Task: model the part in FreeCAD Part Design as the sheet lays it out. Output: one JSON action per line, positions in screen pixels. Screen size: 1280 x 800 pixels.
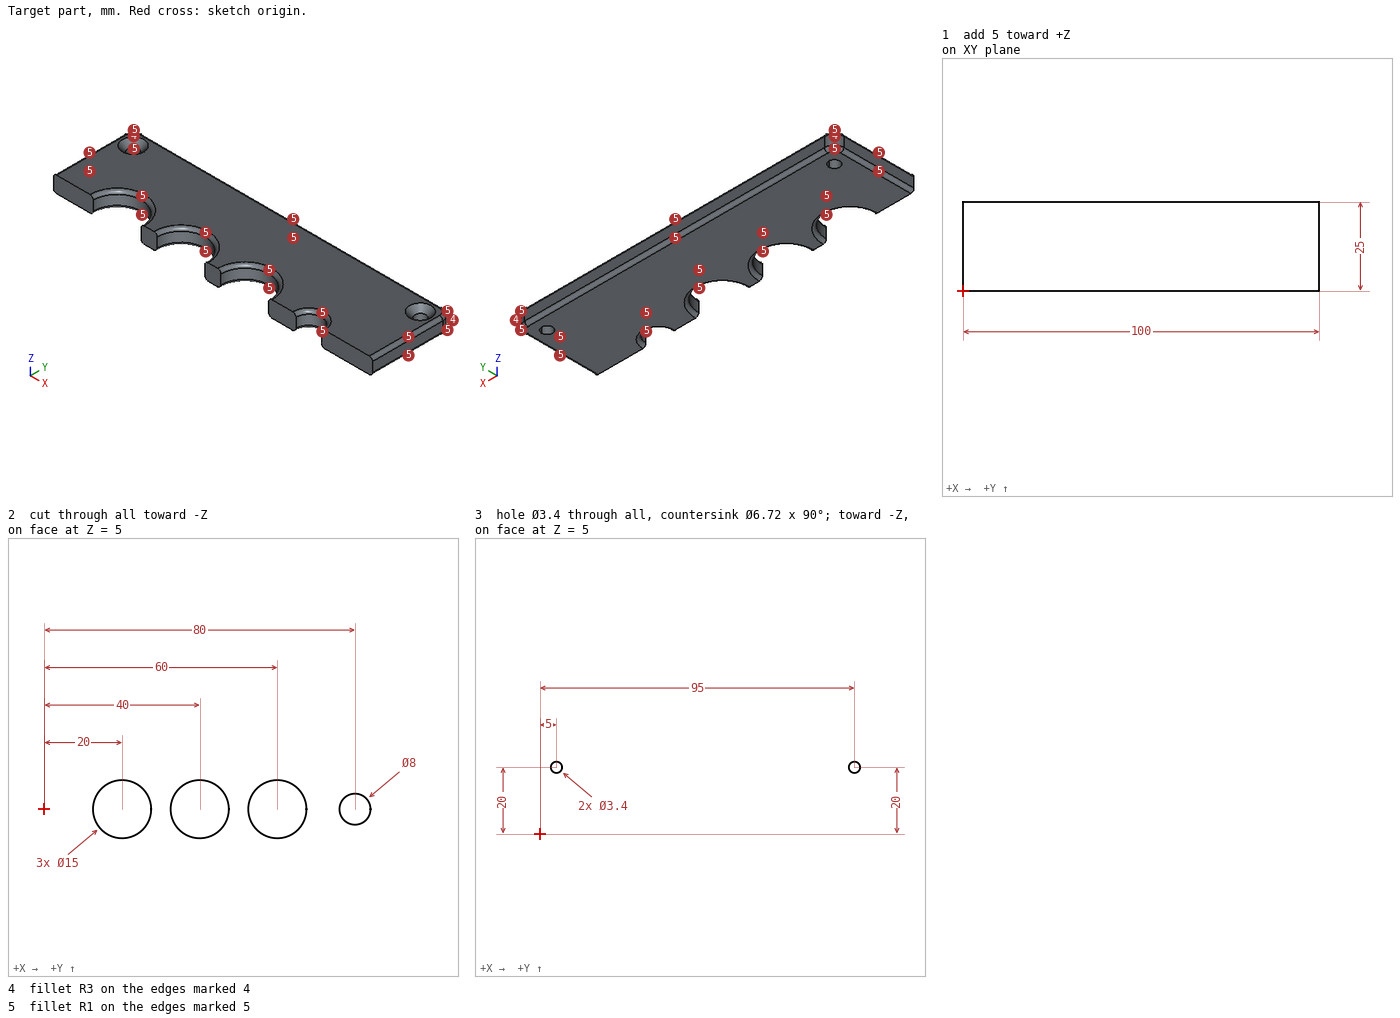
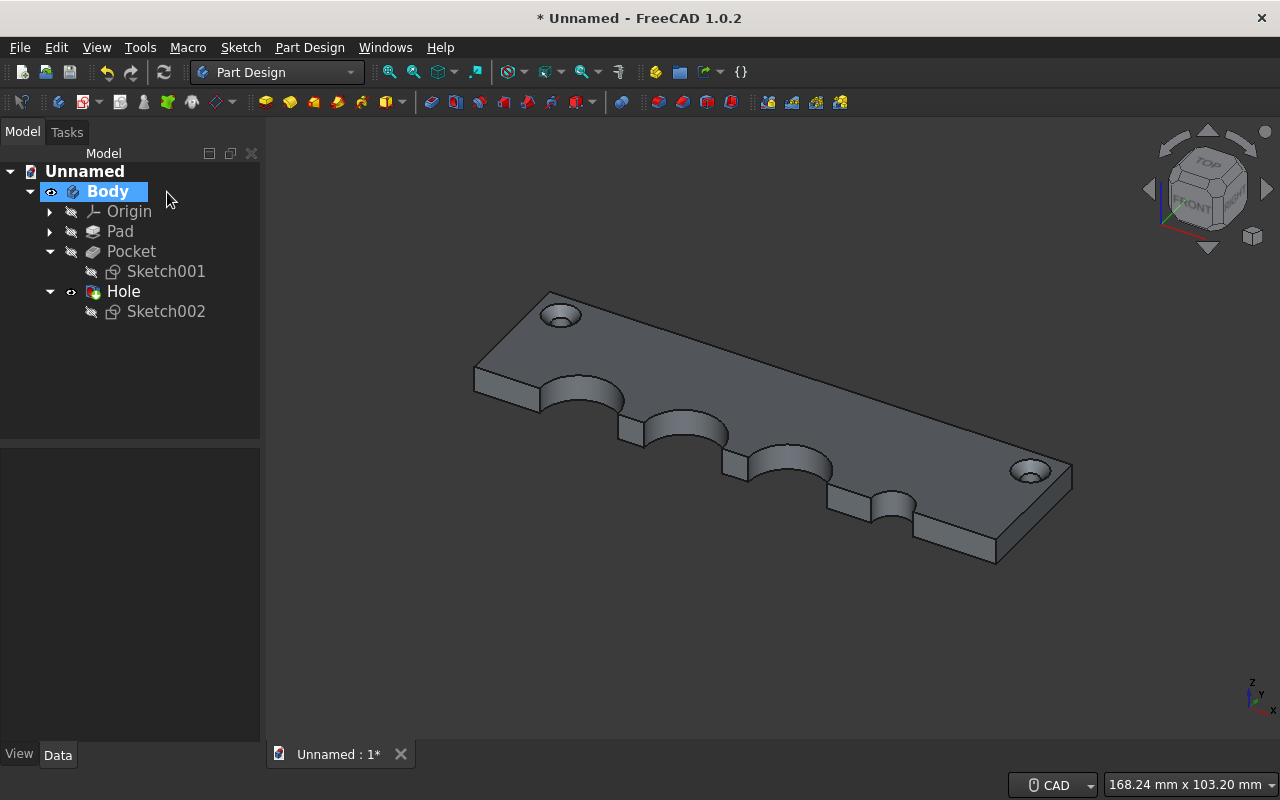
{"action": "key", "text": "0"}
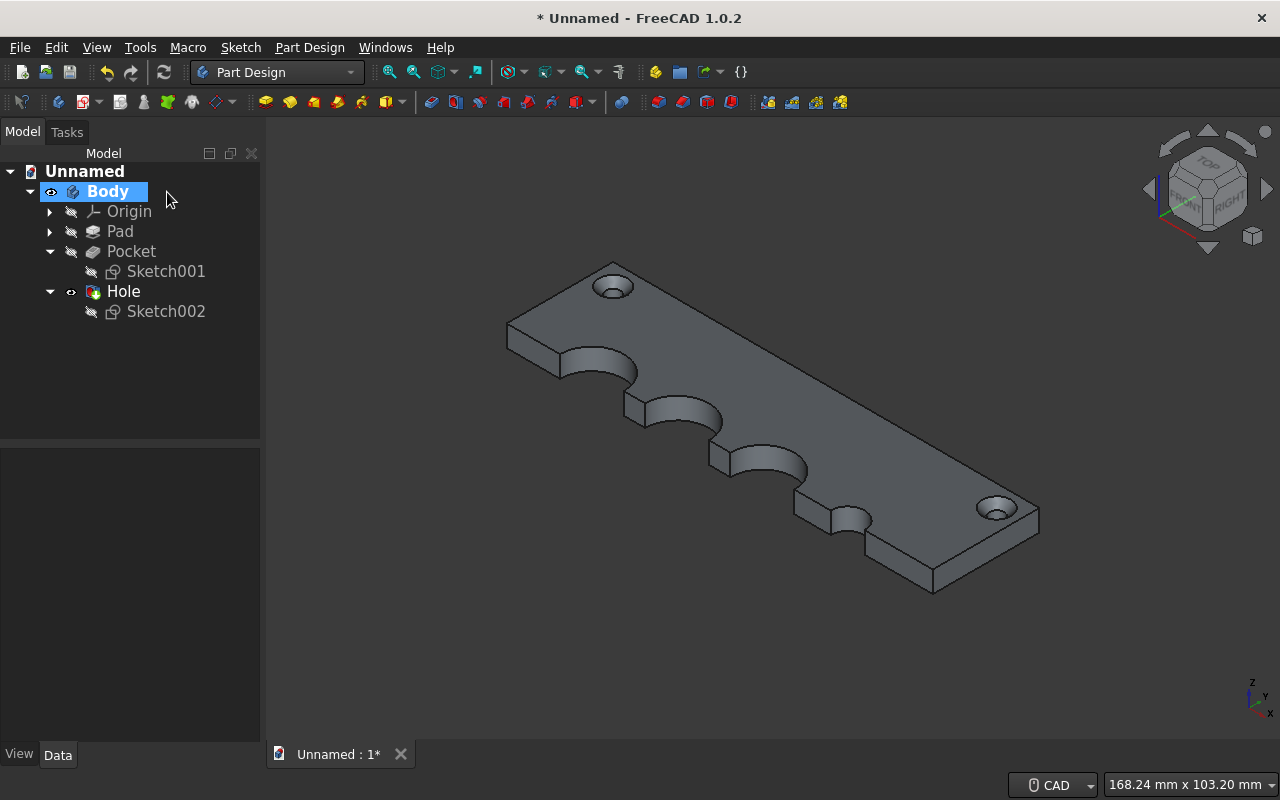
{"action": "key", "text": "2"}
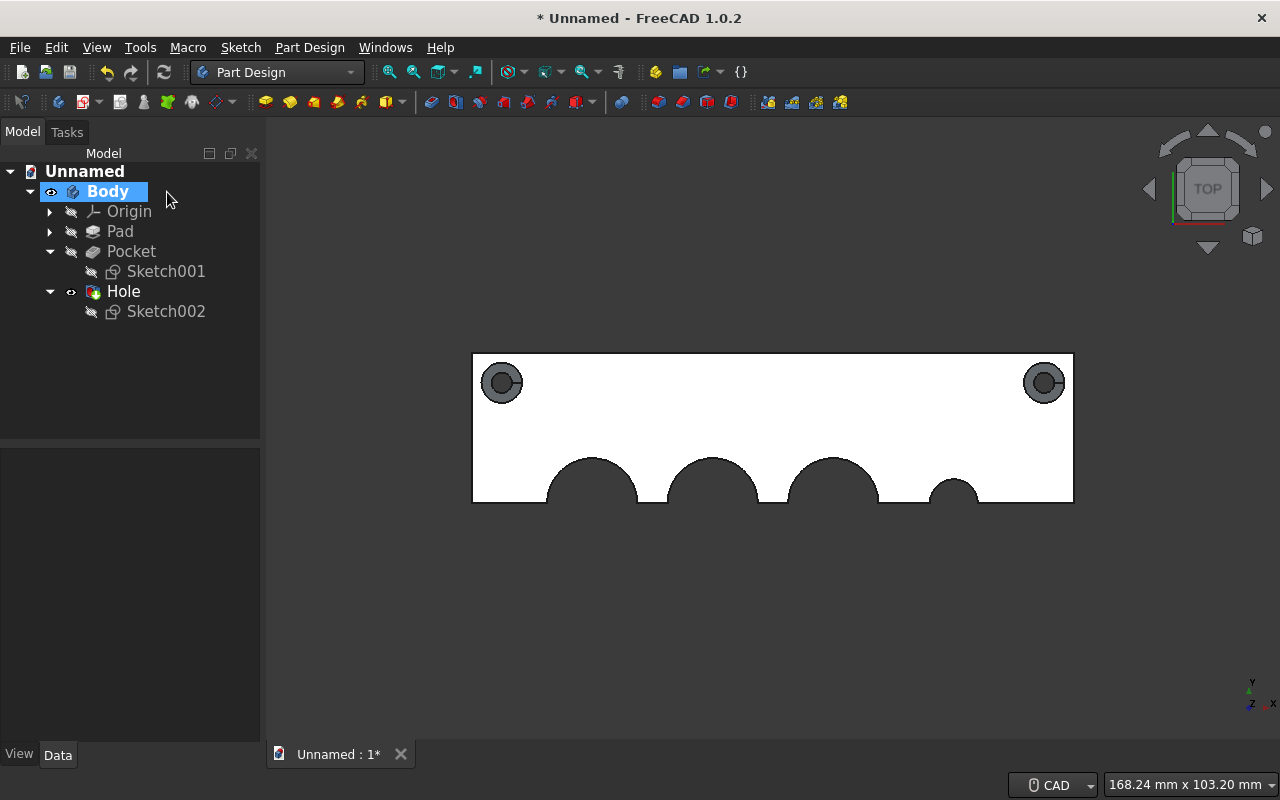
{"action": "key", "text": "1"}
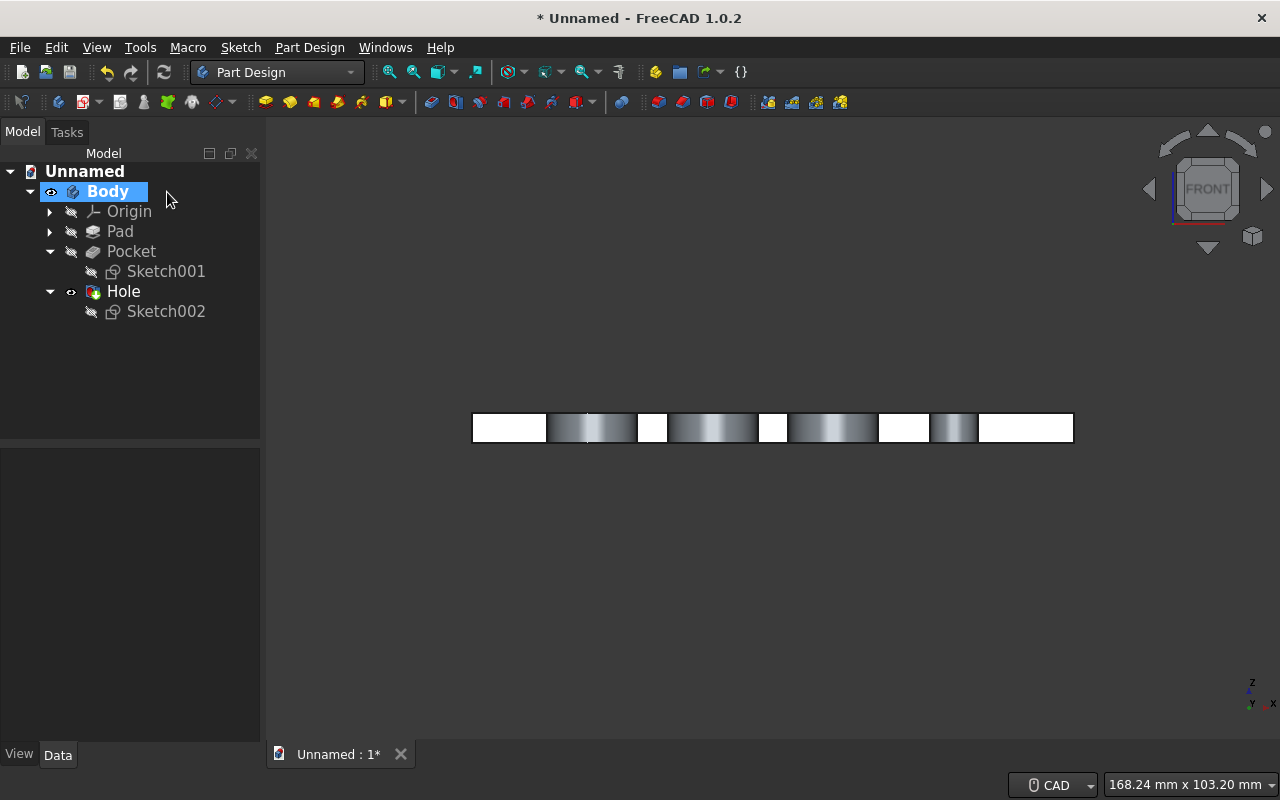
{"action": "key", "text": "3"}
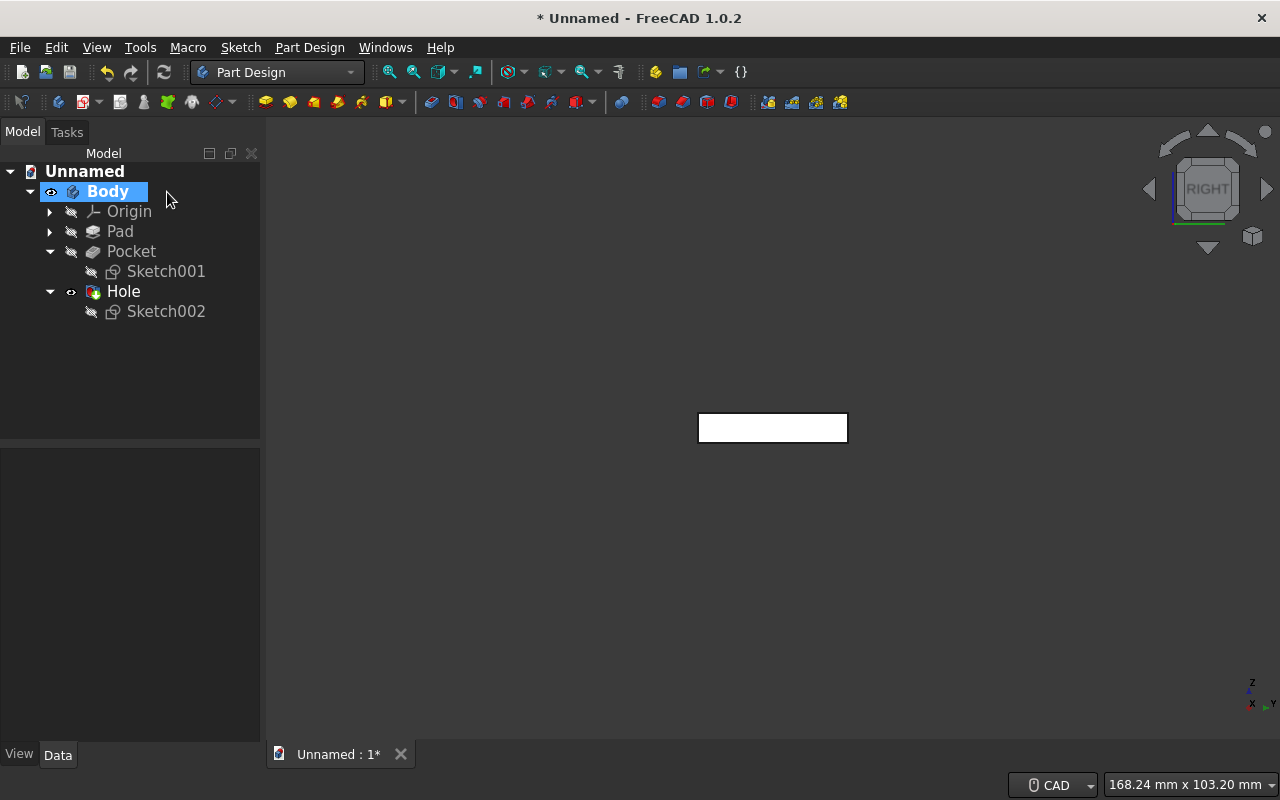
{"action": "left_click", "coordinate": [390, 72]}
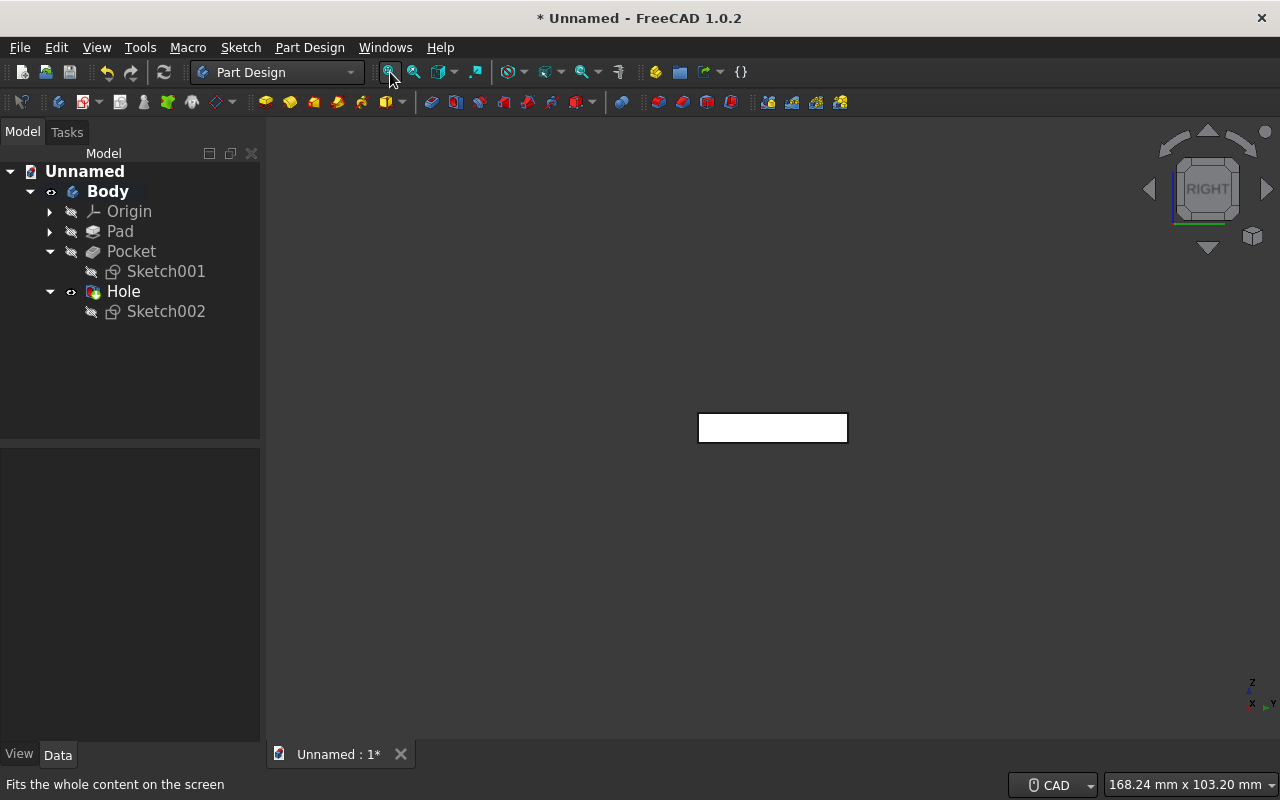
{"action": "left_click", "coordinate": [848, 427]}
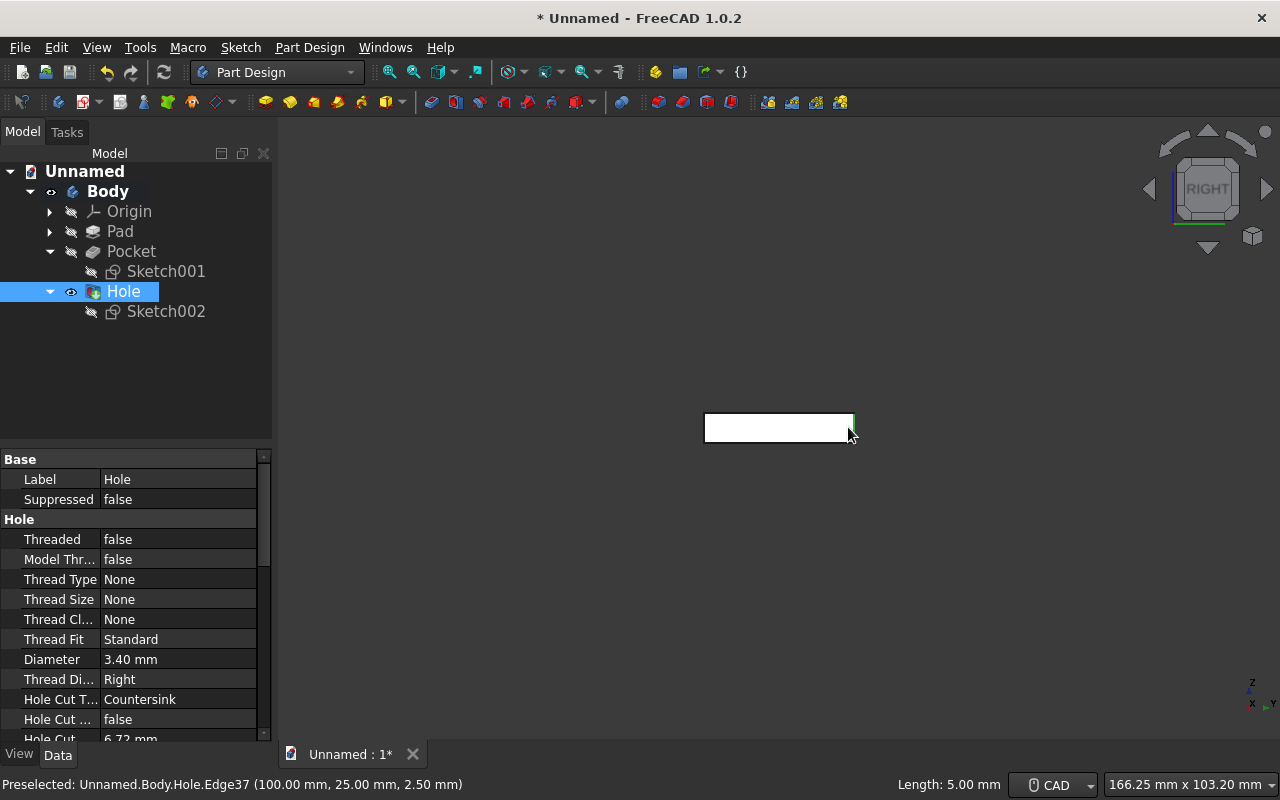
{"action": "key", "text": "5"}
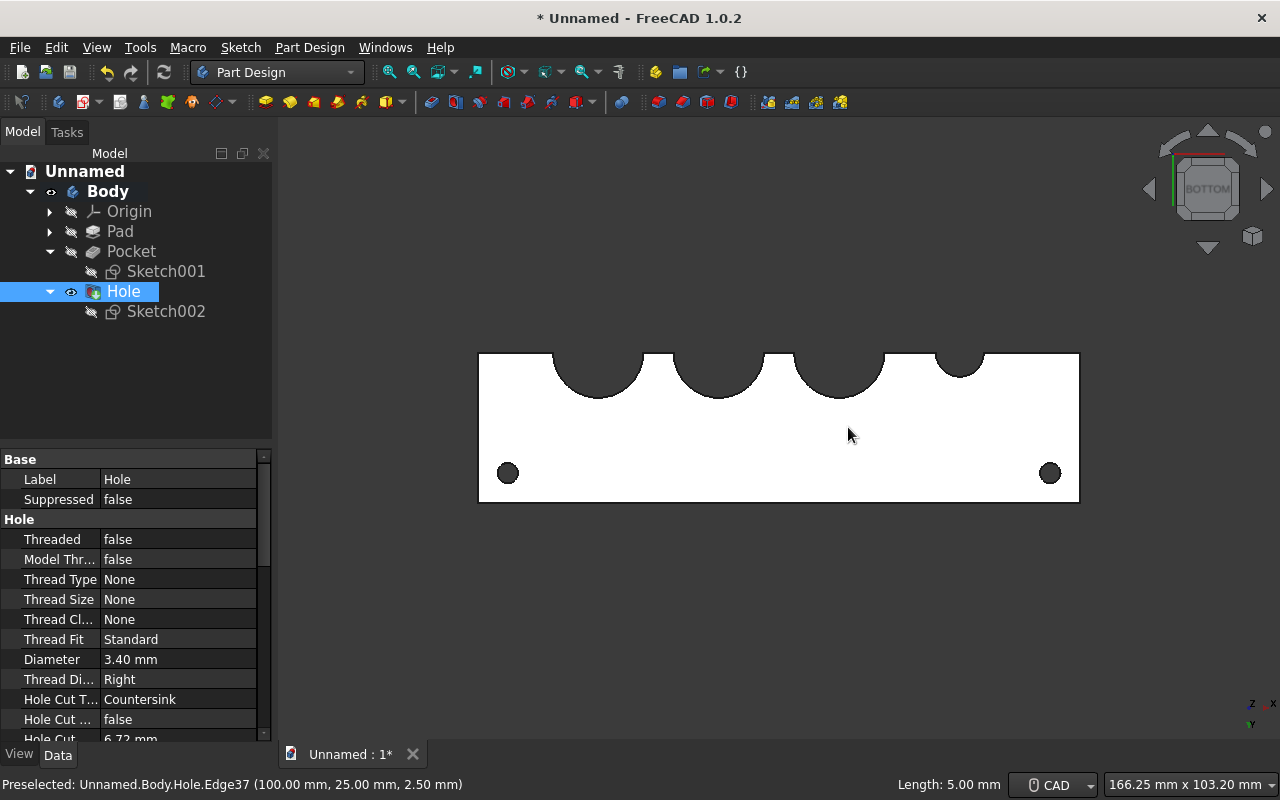
{"action": "key", "text": "4"}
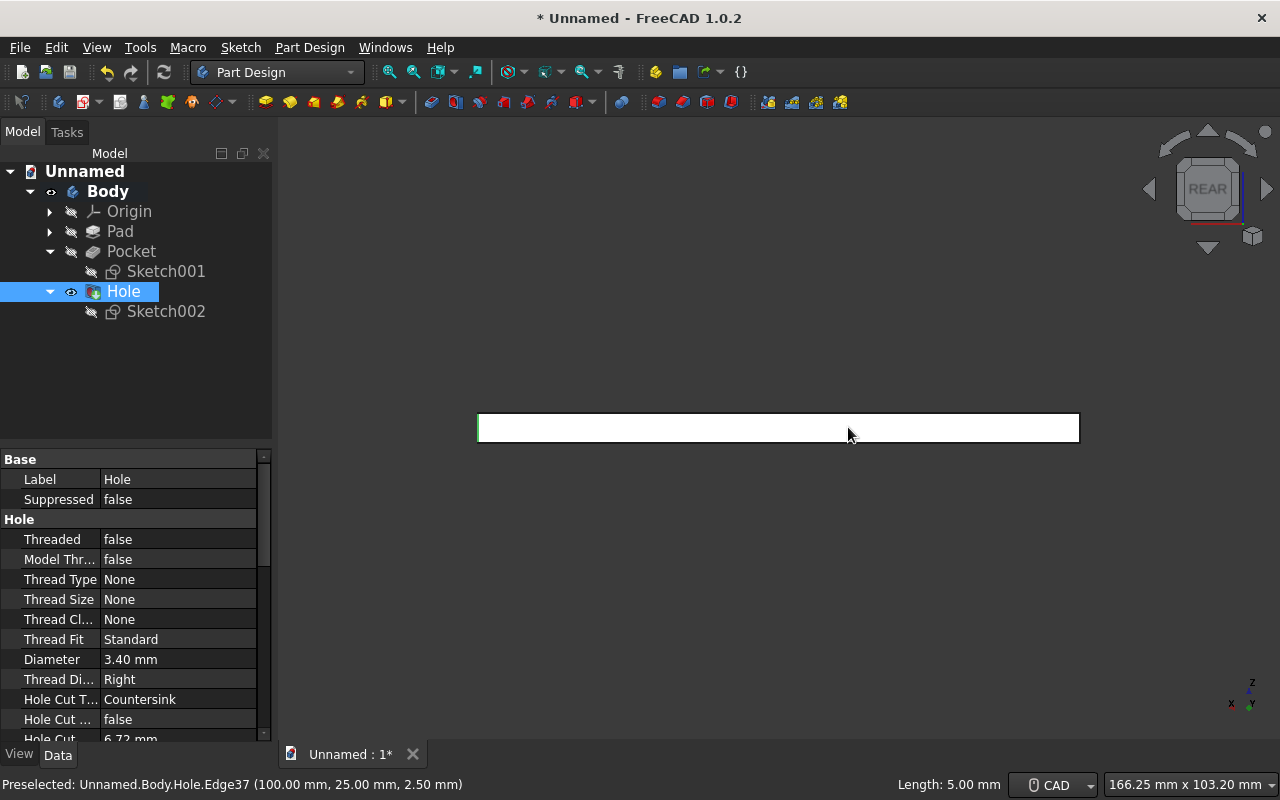
{"action": "left_click", "coordinate": [1080, 427], "text": "ctrl"}